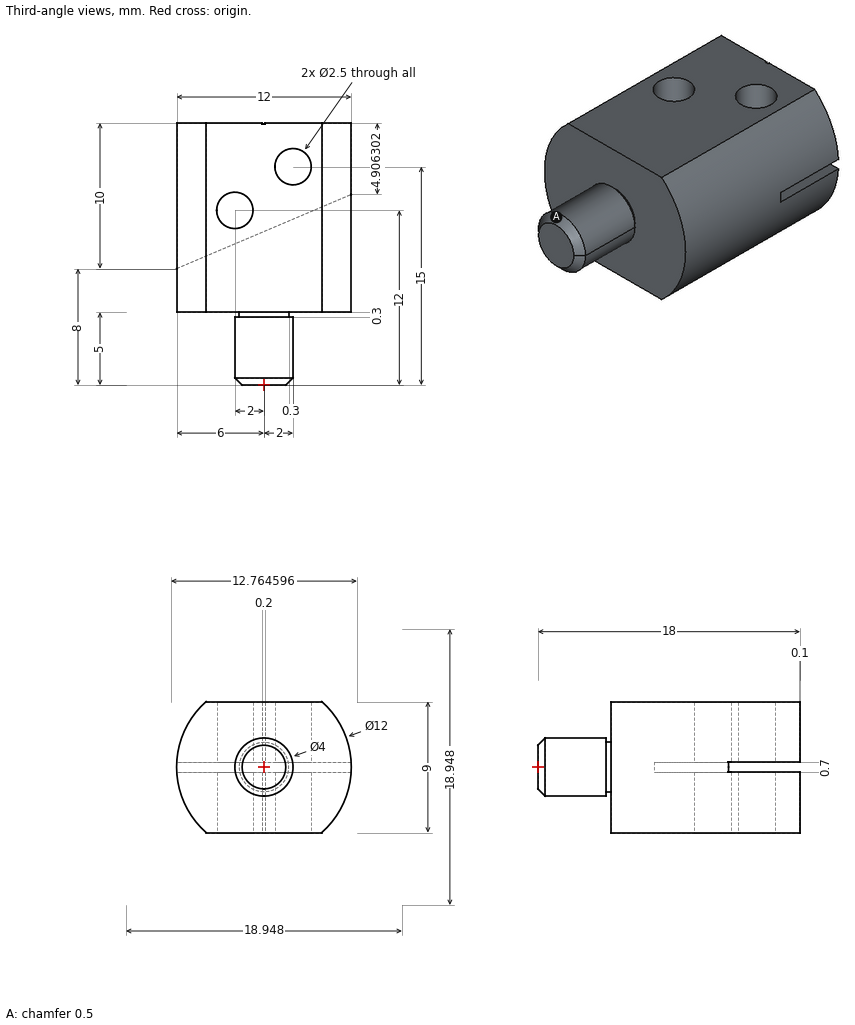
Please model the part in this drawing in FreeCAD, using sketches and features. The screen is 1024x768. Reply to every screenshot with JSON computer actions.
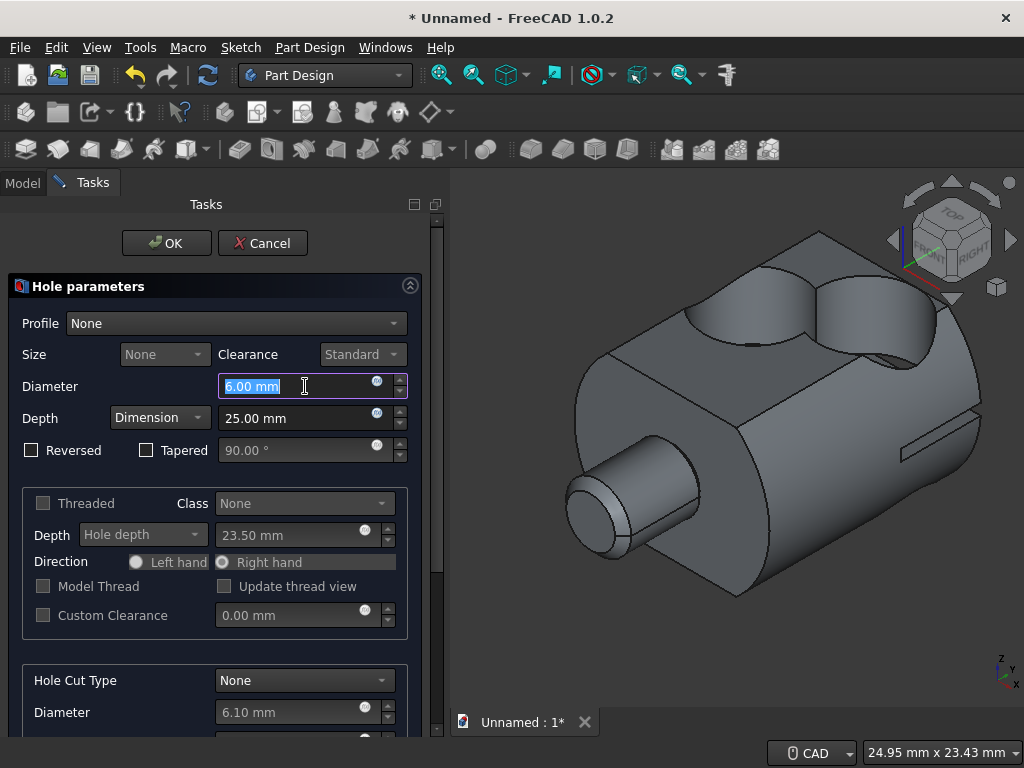
{"action": "type", "text": "2.5"}
{"action": "key", "text": "Tab"}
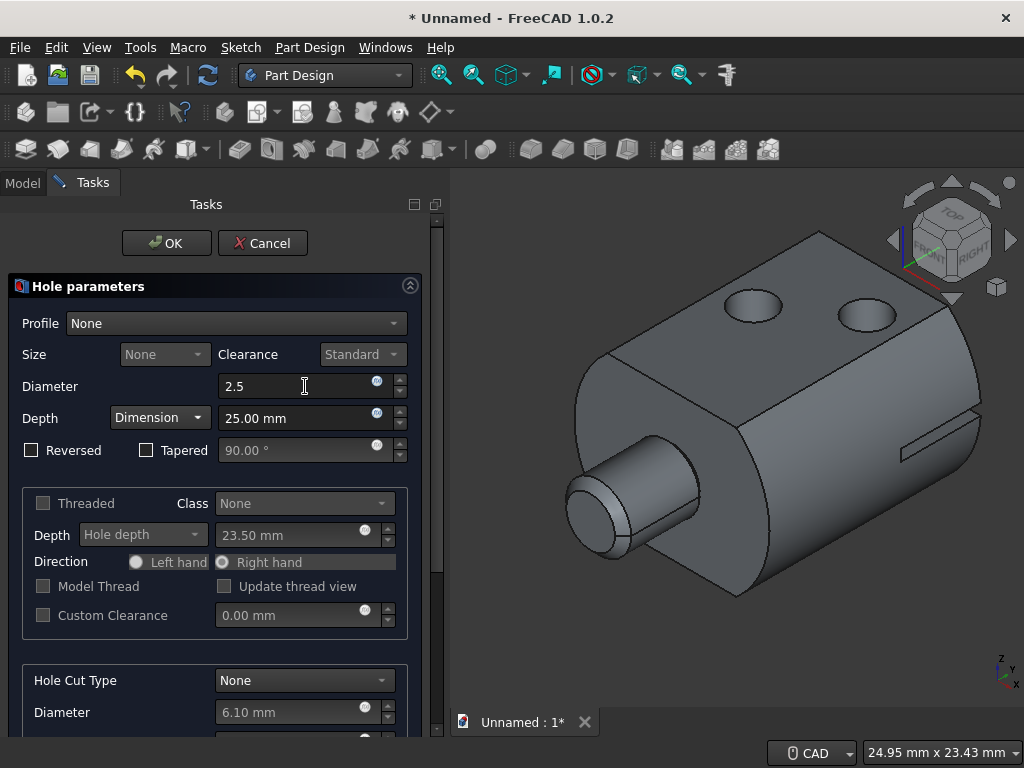
{"action": "left_click", "coordinate": [161, 418]}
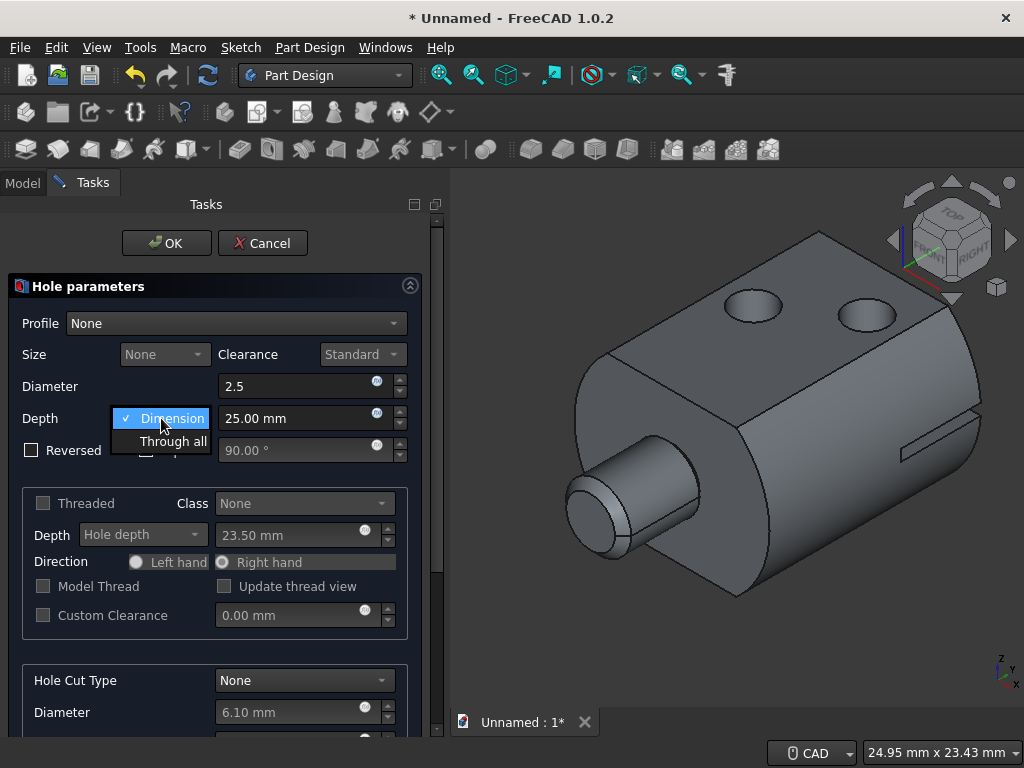
{"action": "left_click", "coordinate": [160, 442]}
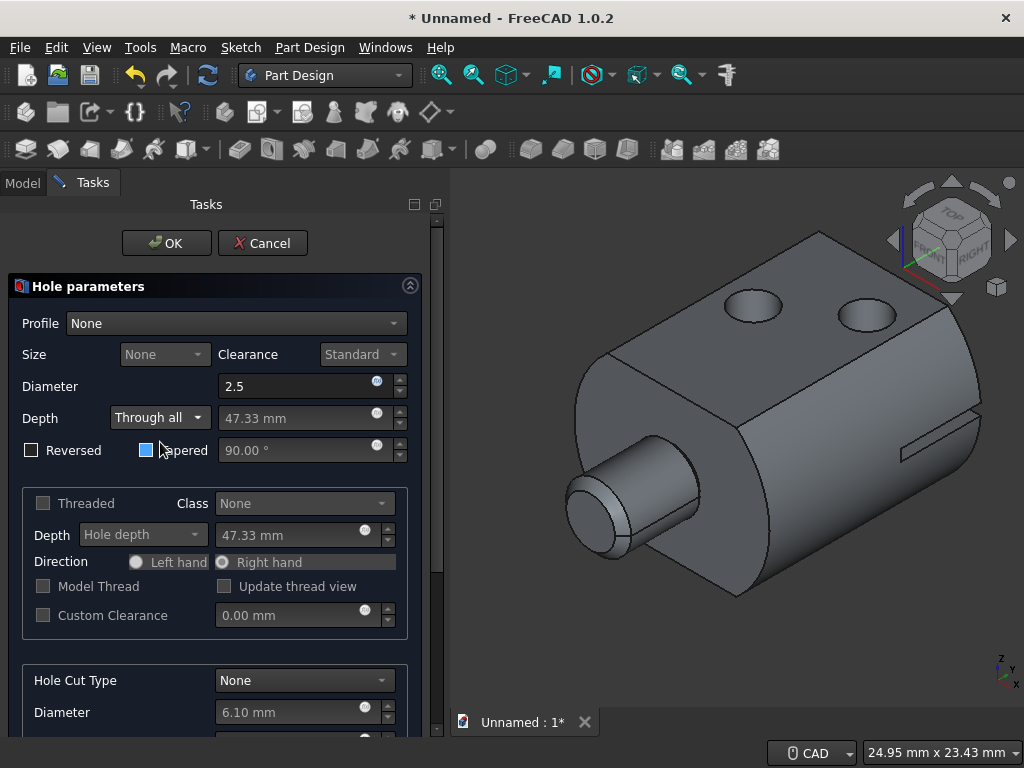
{"action": "left_click", "coordinate": [167, 243]}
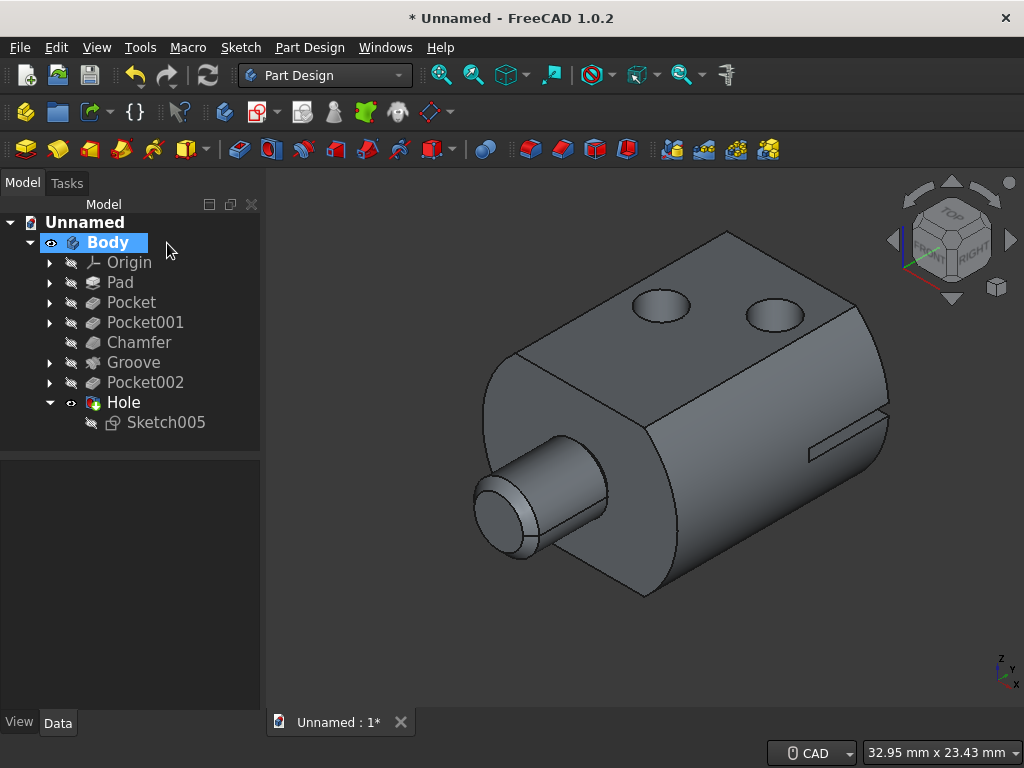
{"action": "key", "text": "4"}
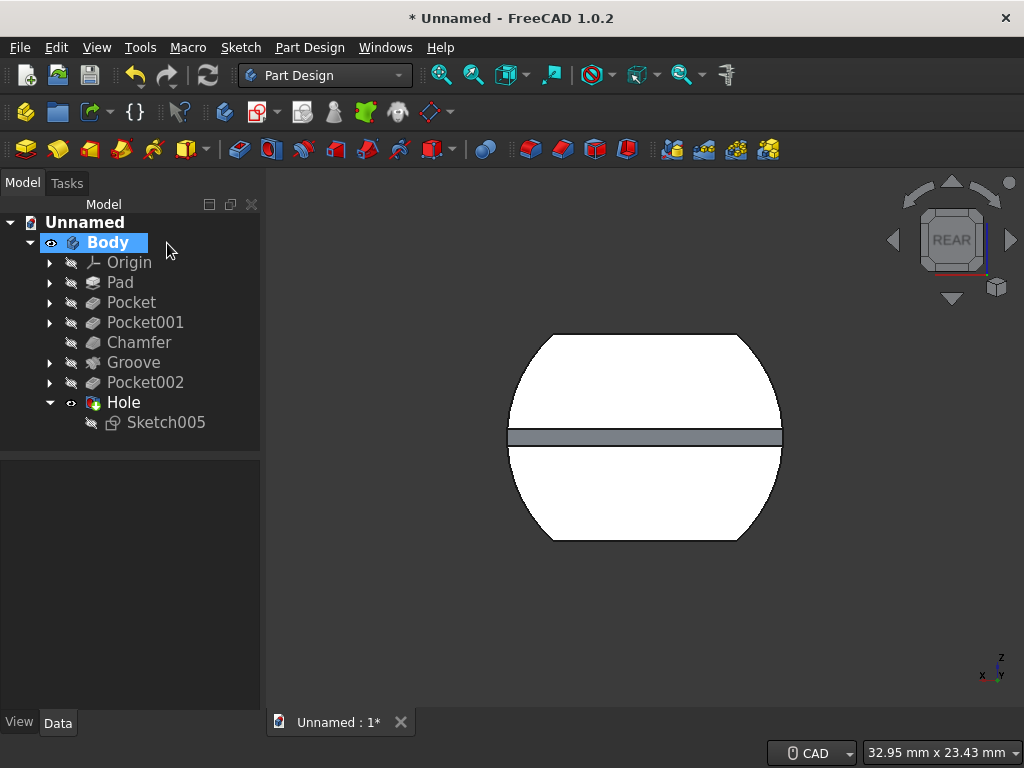
{"action": "key", "text": "v f"}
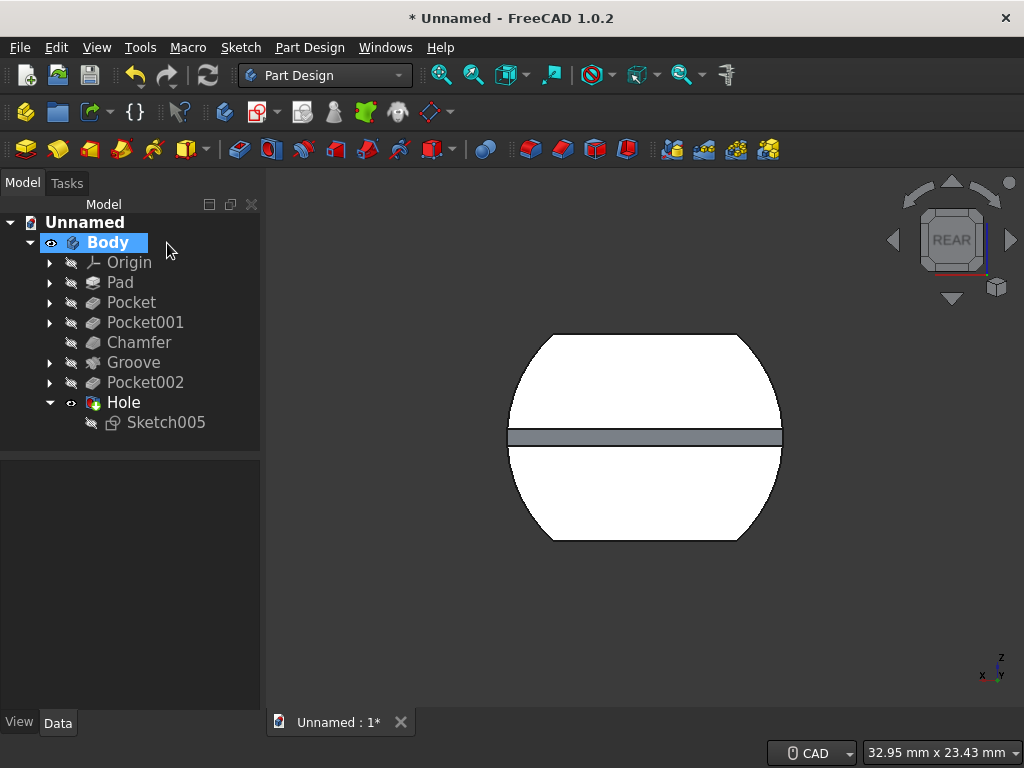
{"action": "left_click", "coordinate": [606, 492]}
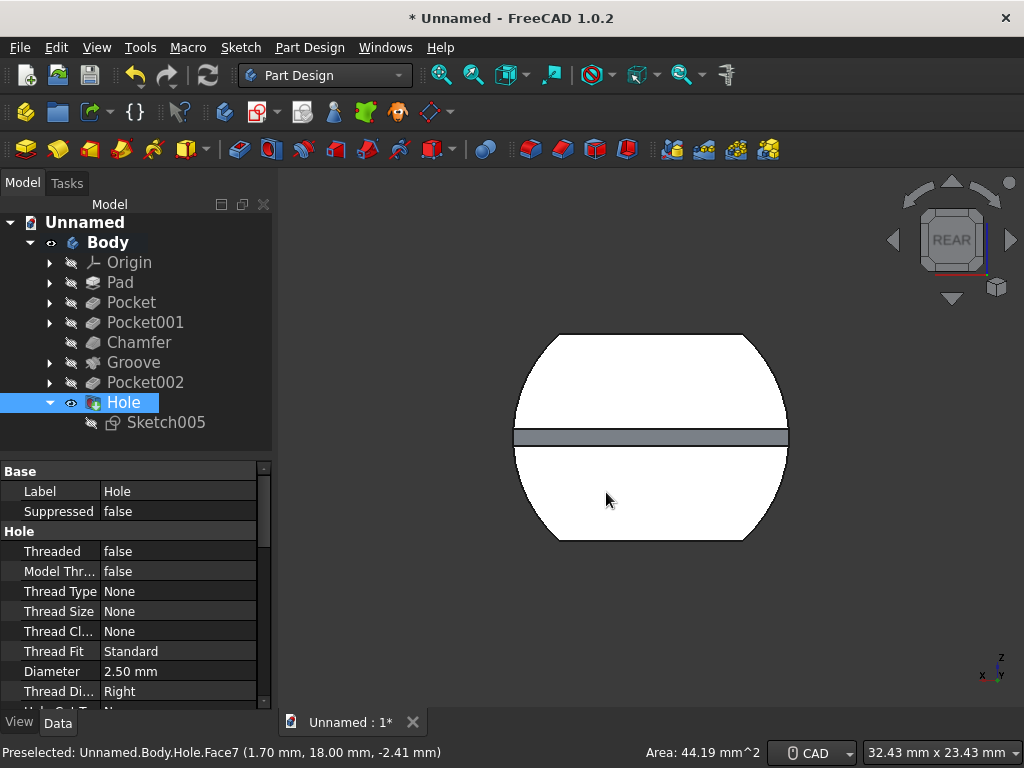
{"action": "left_click", "coordinate": [258, 112]}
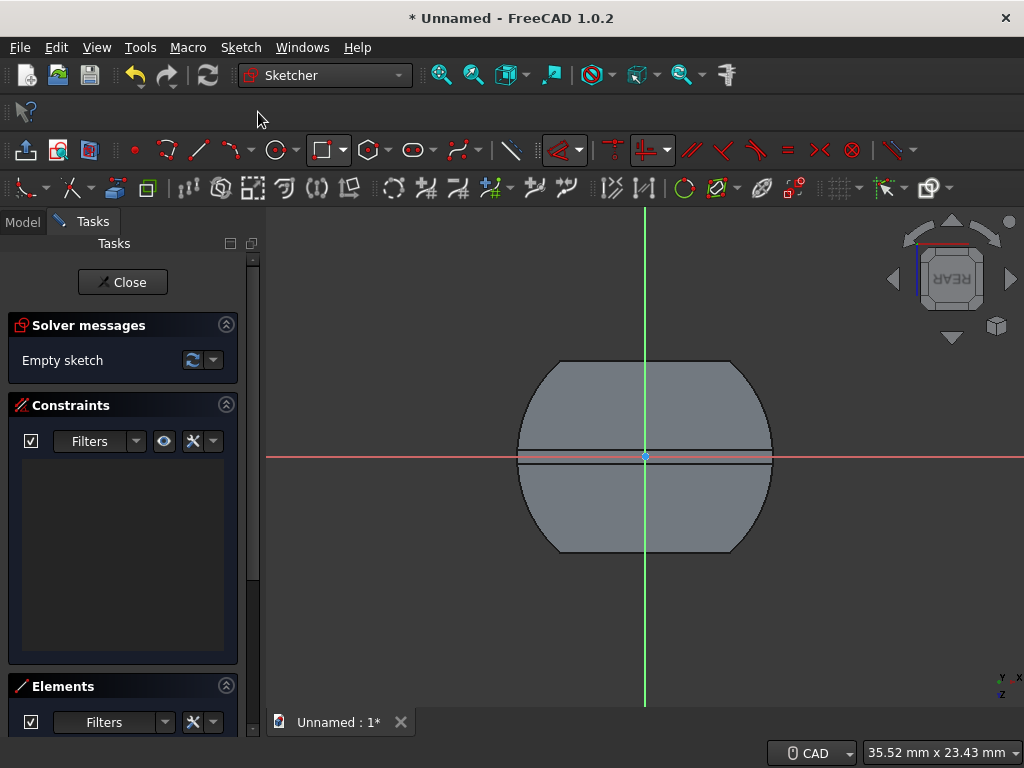
{"action": "scroll", "coordinate": [784, 457], "scroll_direction": "up", "scroll_amount": 2}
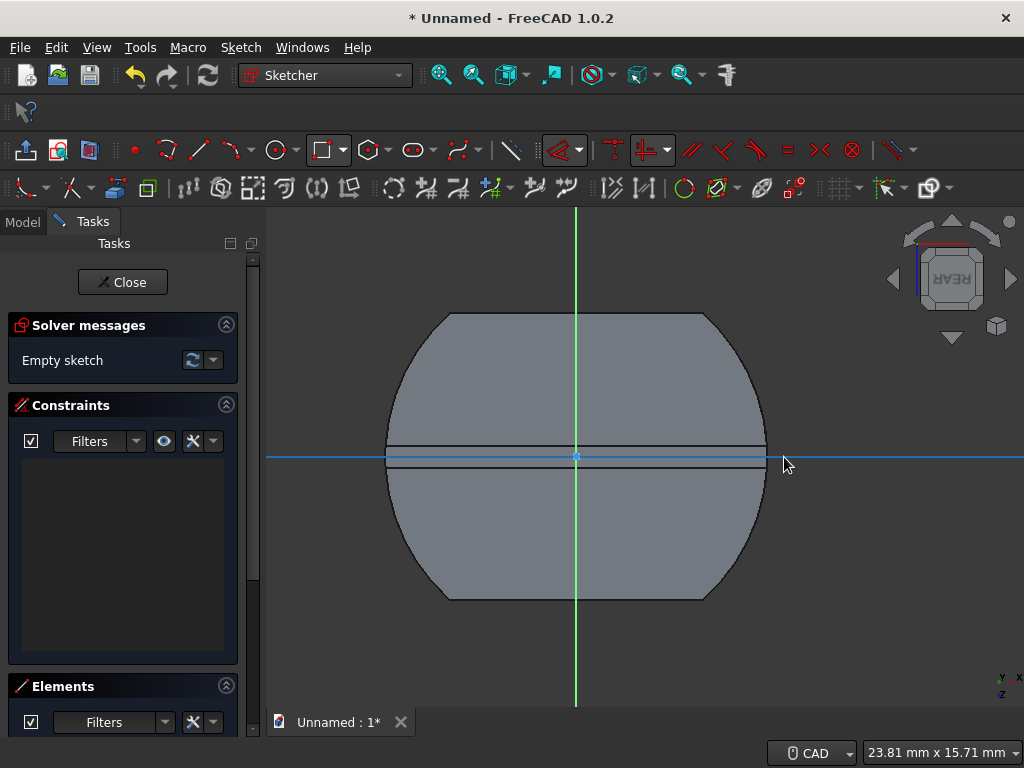
{"action": "key", "text": "g v"}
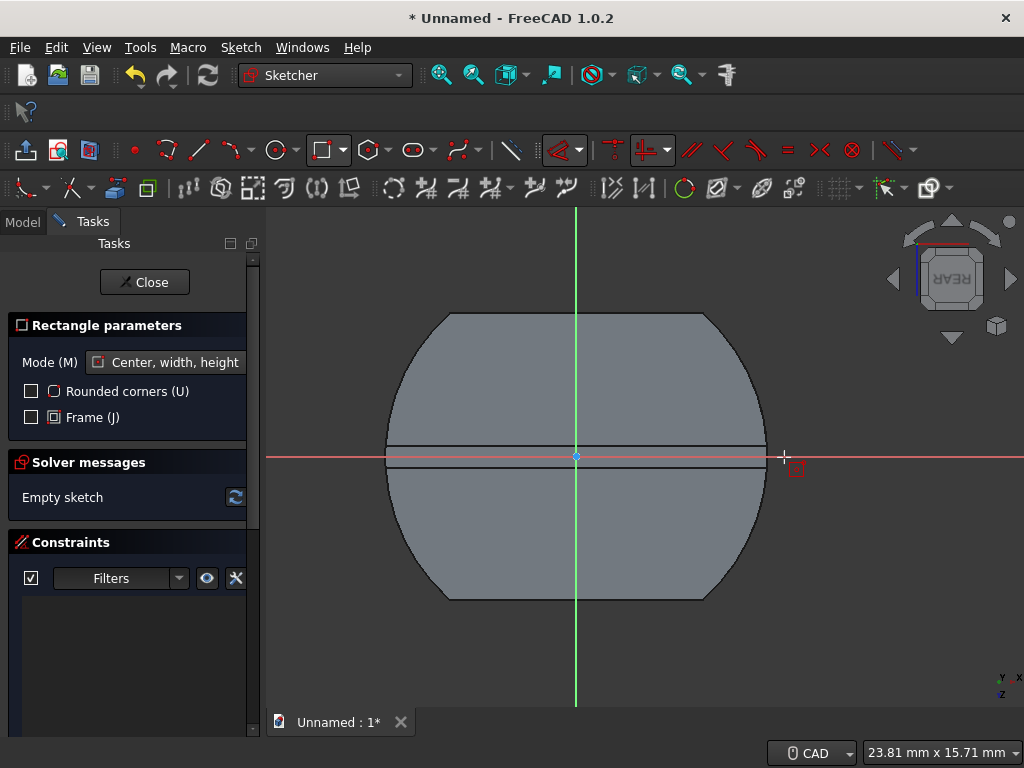
{"action": "scroll", "coordinate": [576, 457], "scroll_direction": "up", "scroll_amount": 9}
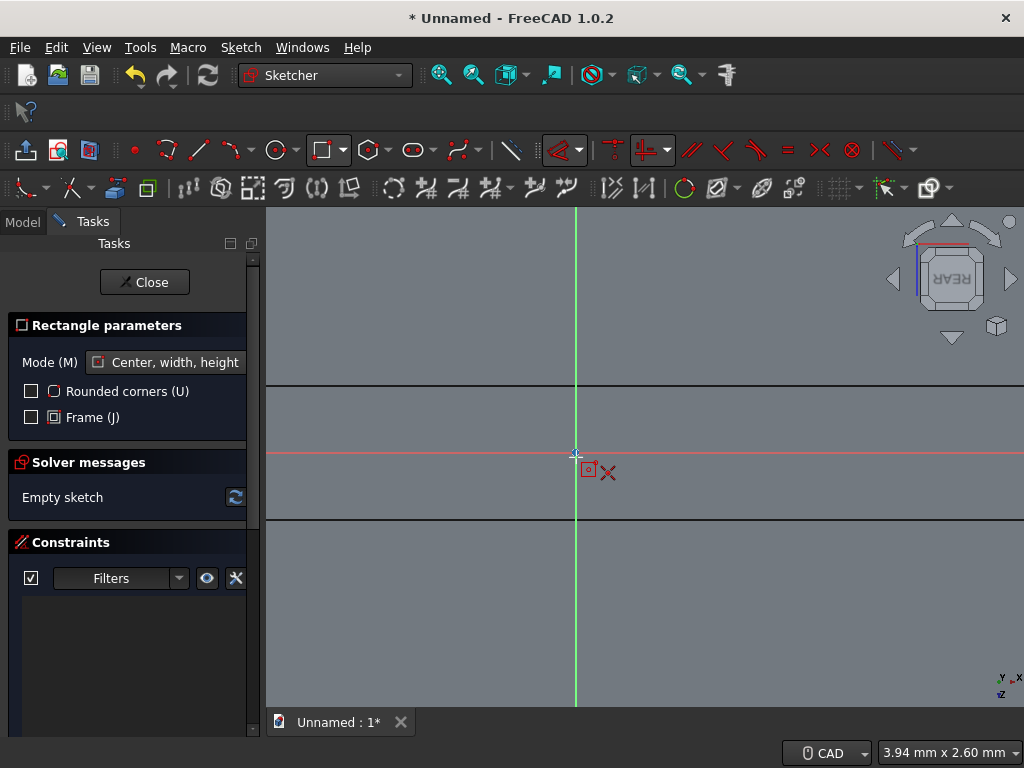
{"action": "scroll", "coordinate": [577, 458], "scroll_direction": "down", "scroll_amount": 9}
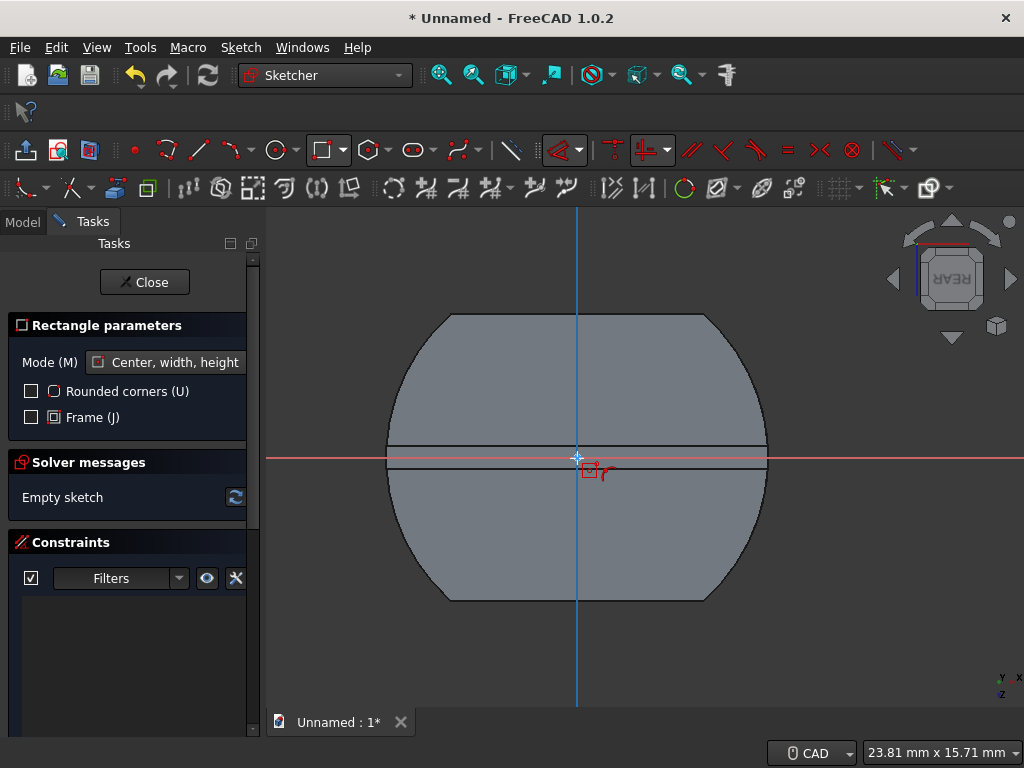
{"action": "left_click", "coordinate": [577, 458]}